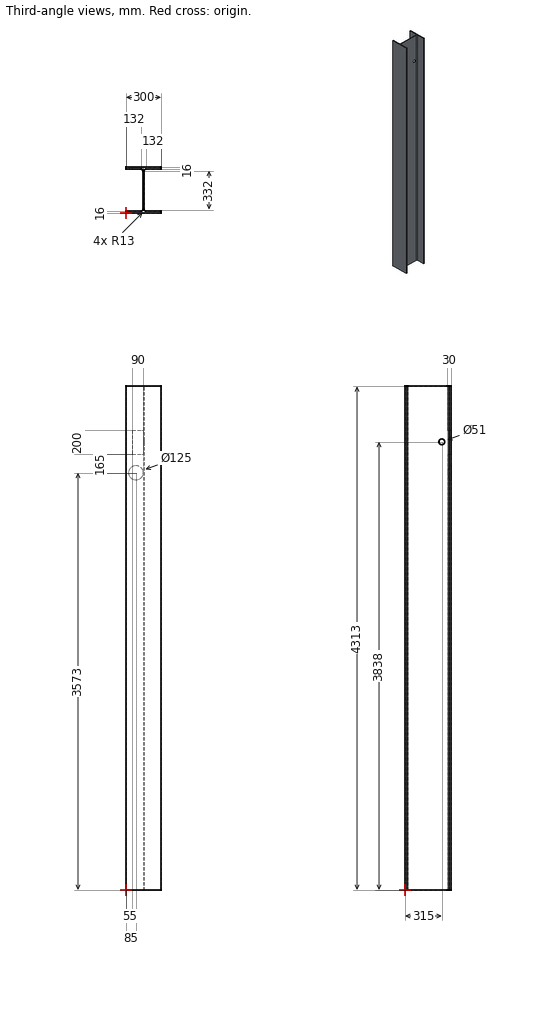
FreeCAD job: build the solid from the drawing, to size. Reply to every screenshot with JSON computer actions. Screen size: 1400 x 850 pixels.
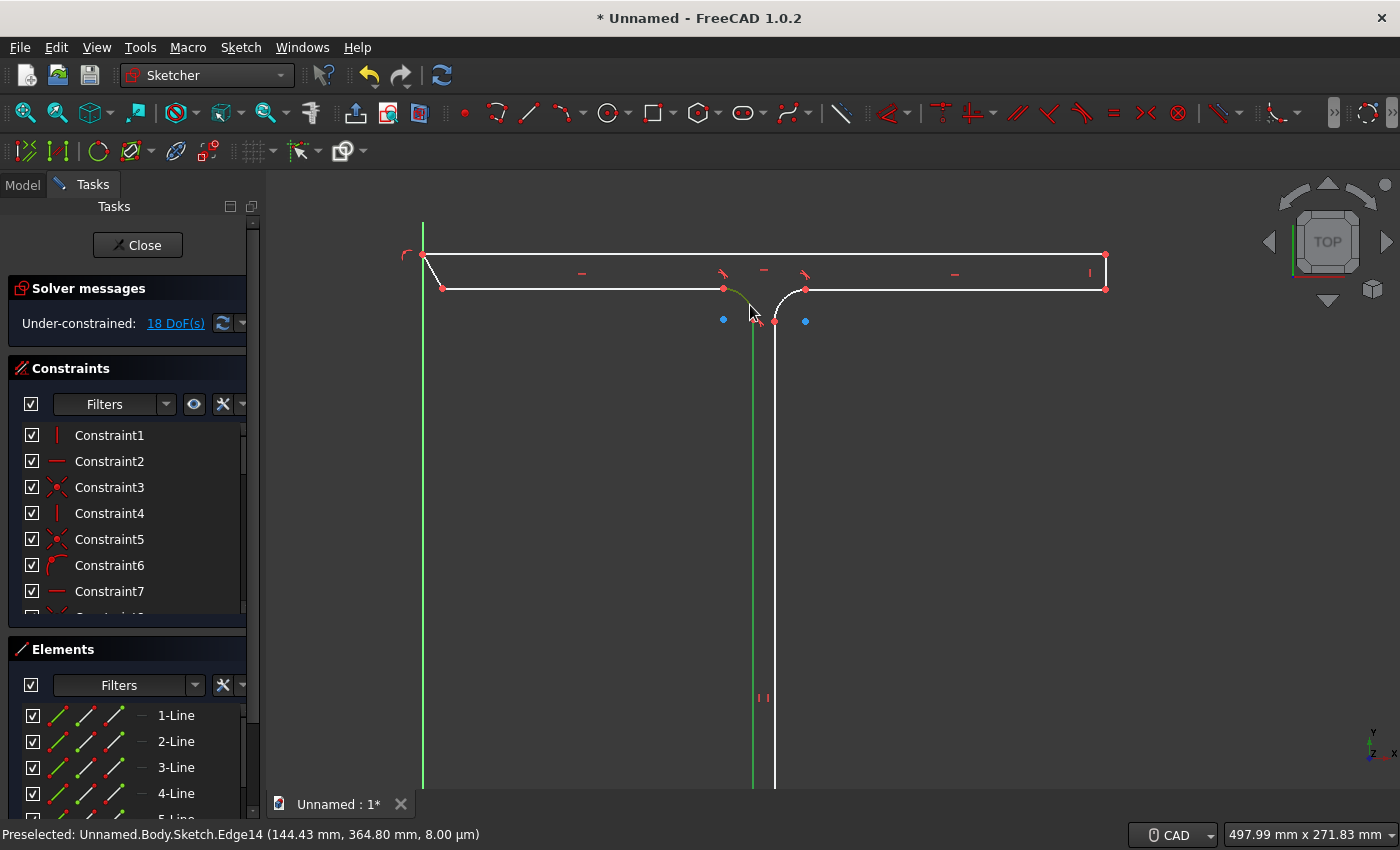
{"action": "left_click", "coordinate": [1082, 114]}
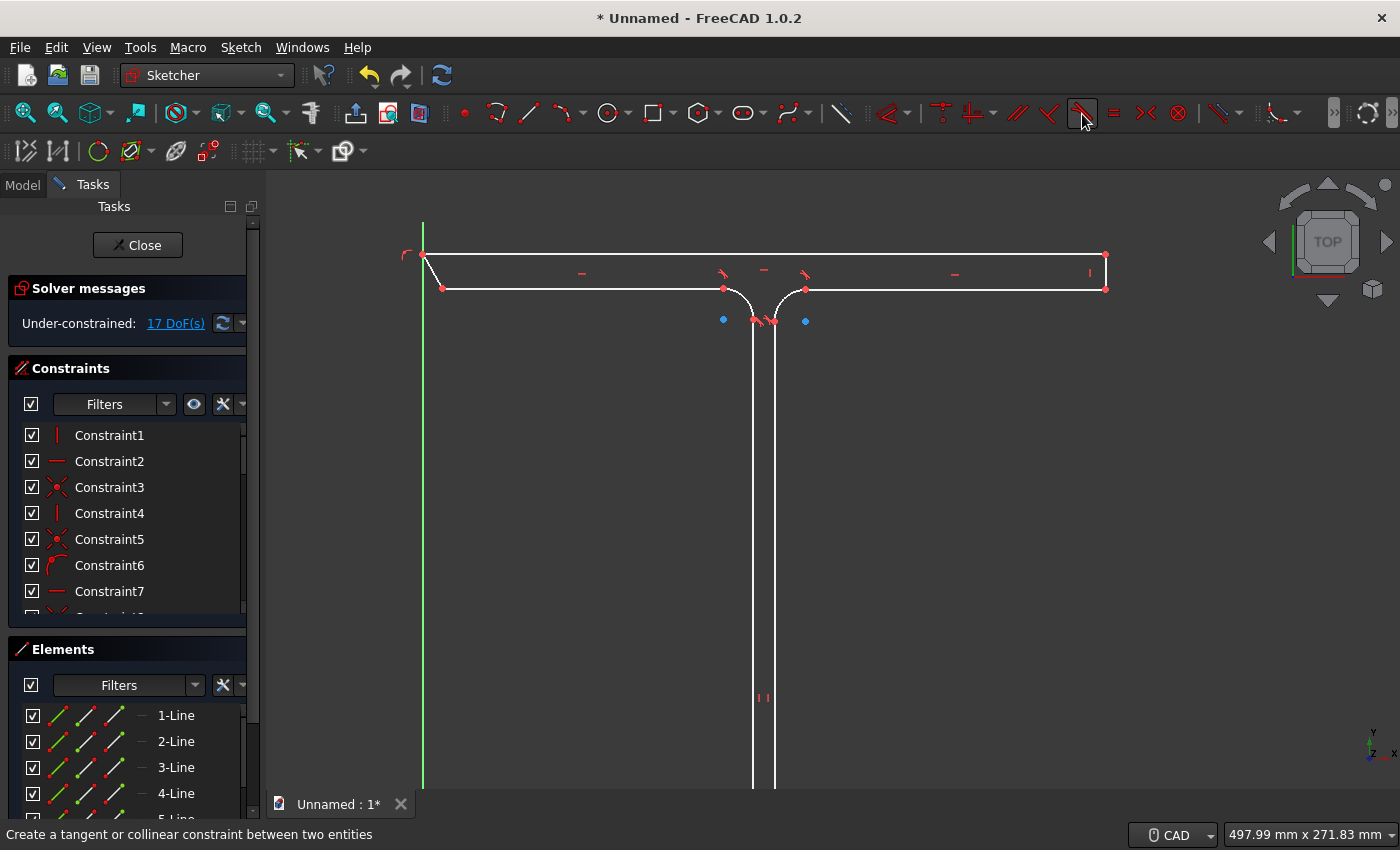
{"action": "left_click", "coordinate": [753, 546]}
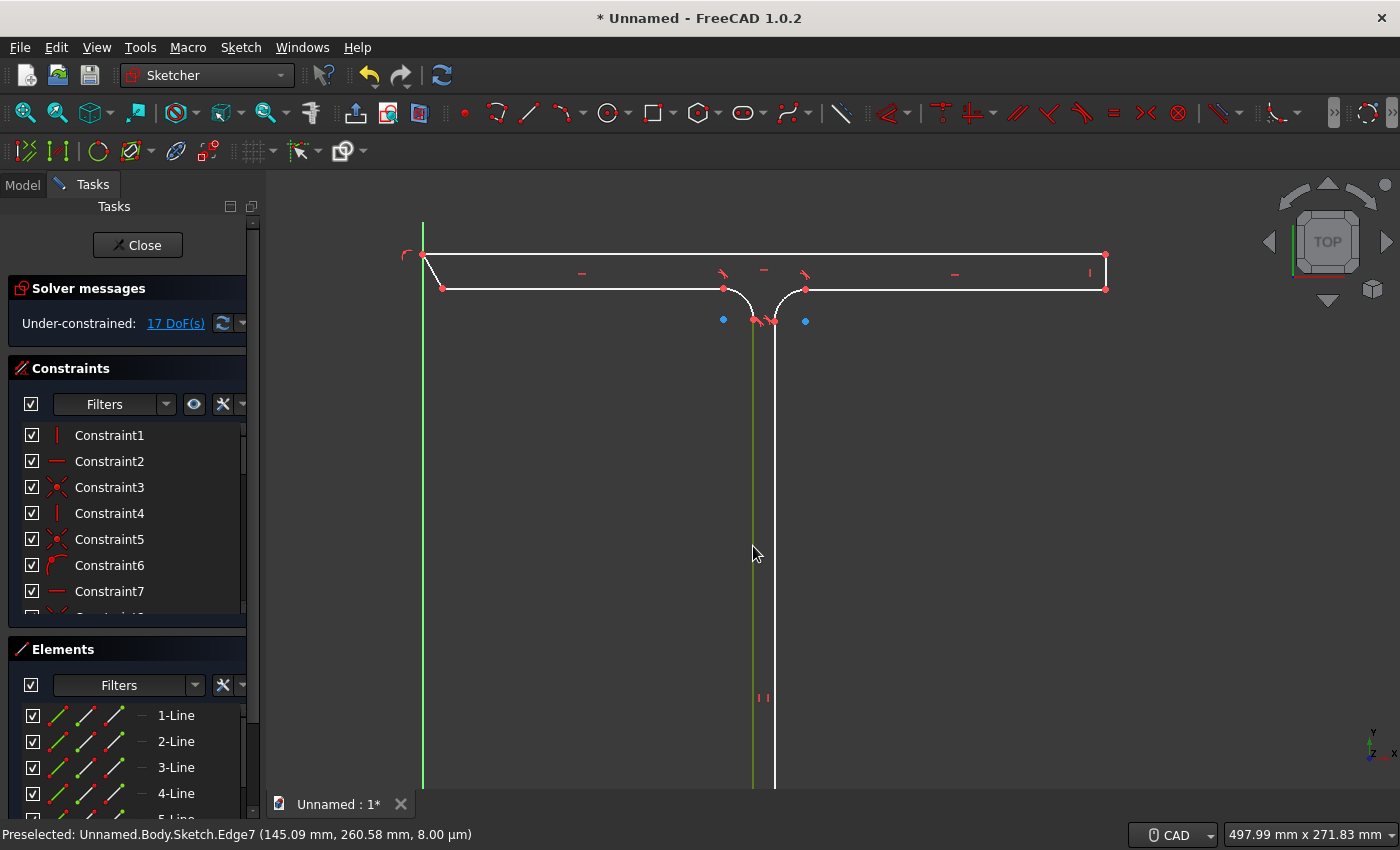
{"action": "scroll", "coordinate": [764, 303], "scroll_direction": "down", "scroll_amount": 4}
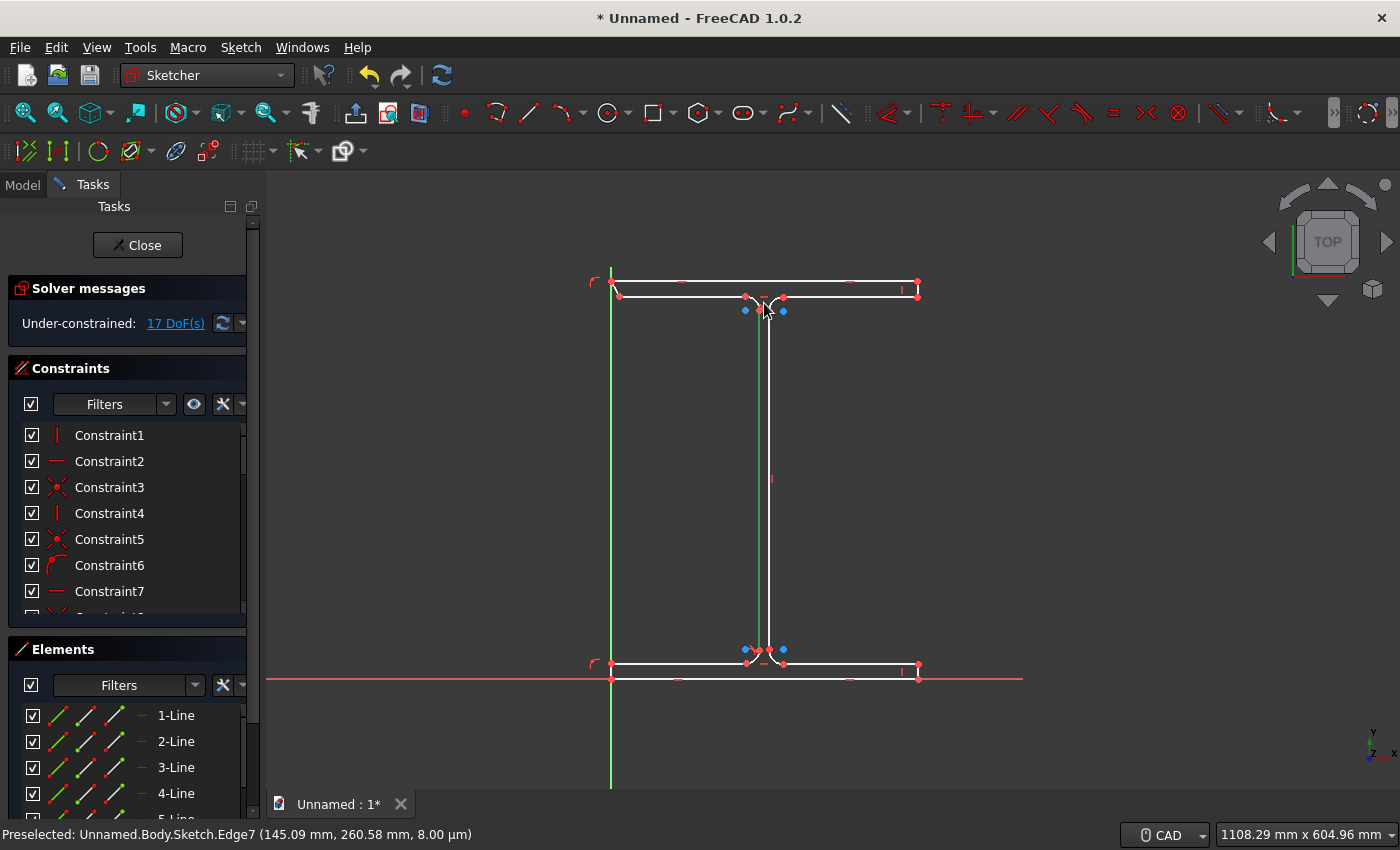
{"action": "scroll", "coordinate": [752, 662], "scroll_direction": "up", "scroll_amount": 5}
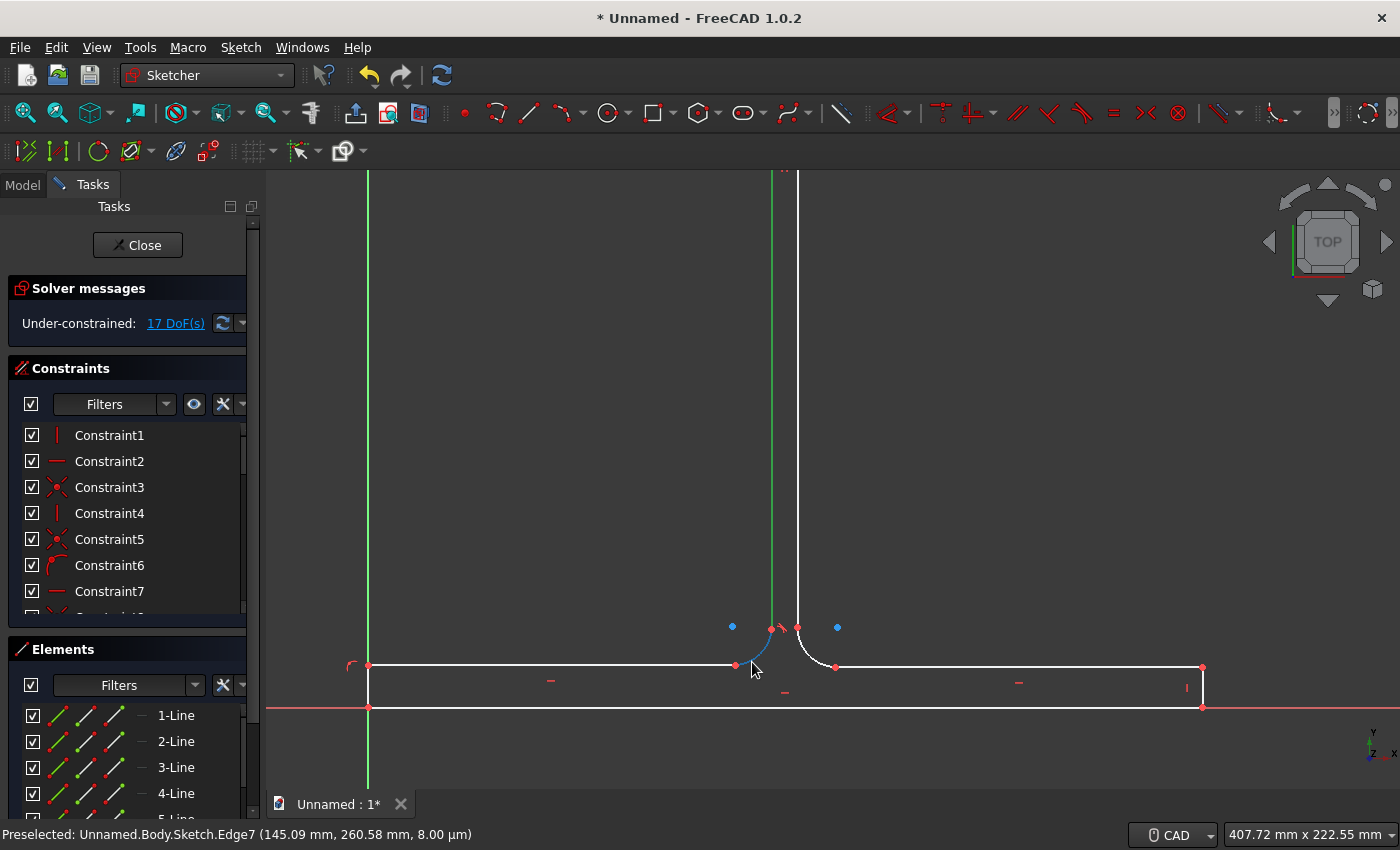
{"action": "left_click", "coordinate": [751, 660]}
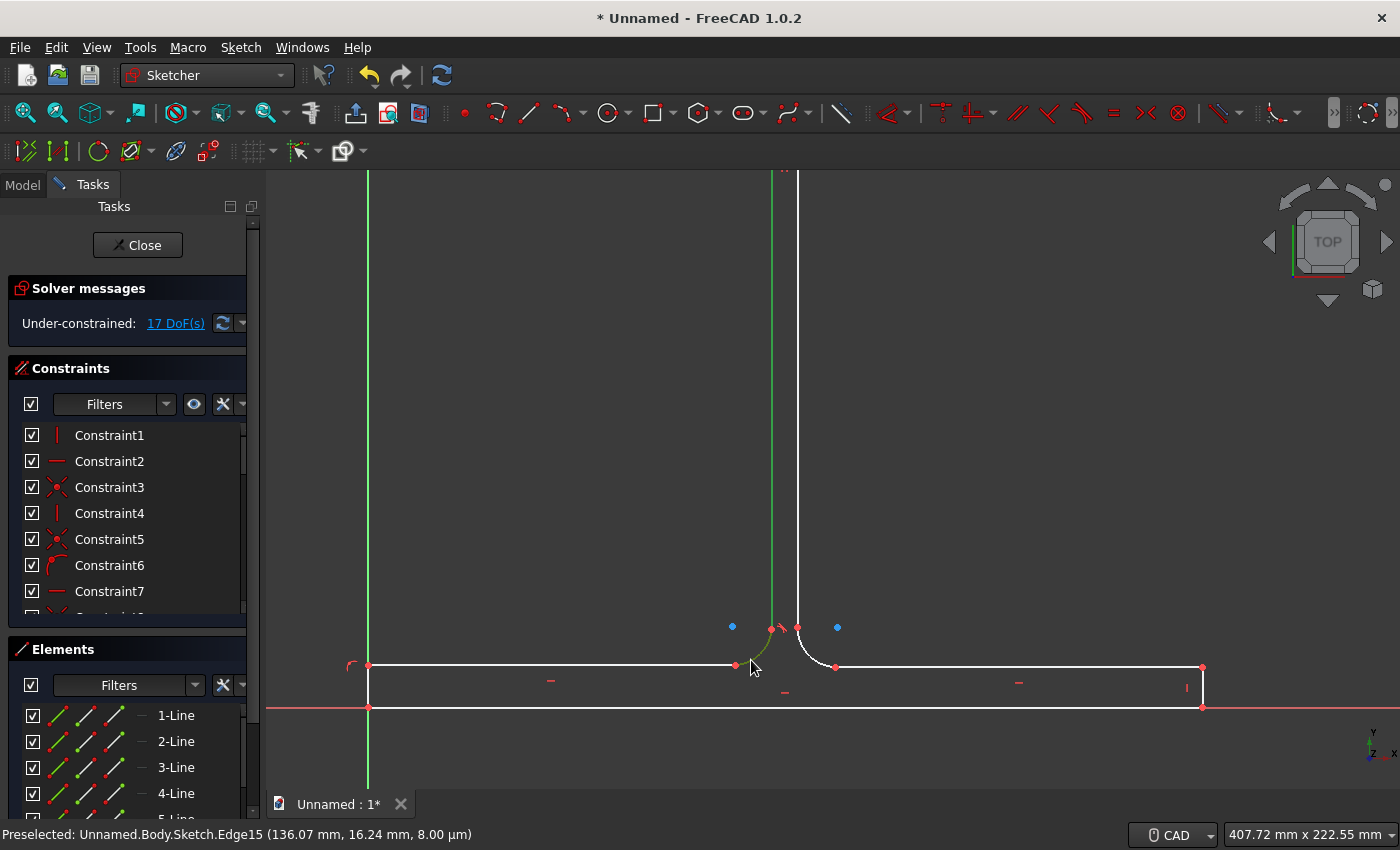
{"action": "left_click", "coordinate": [1082, 114]}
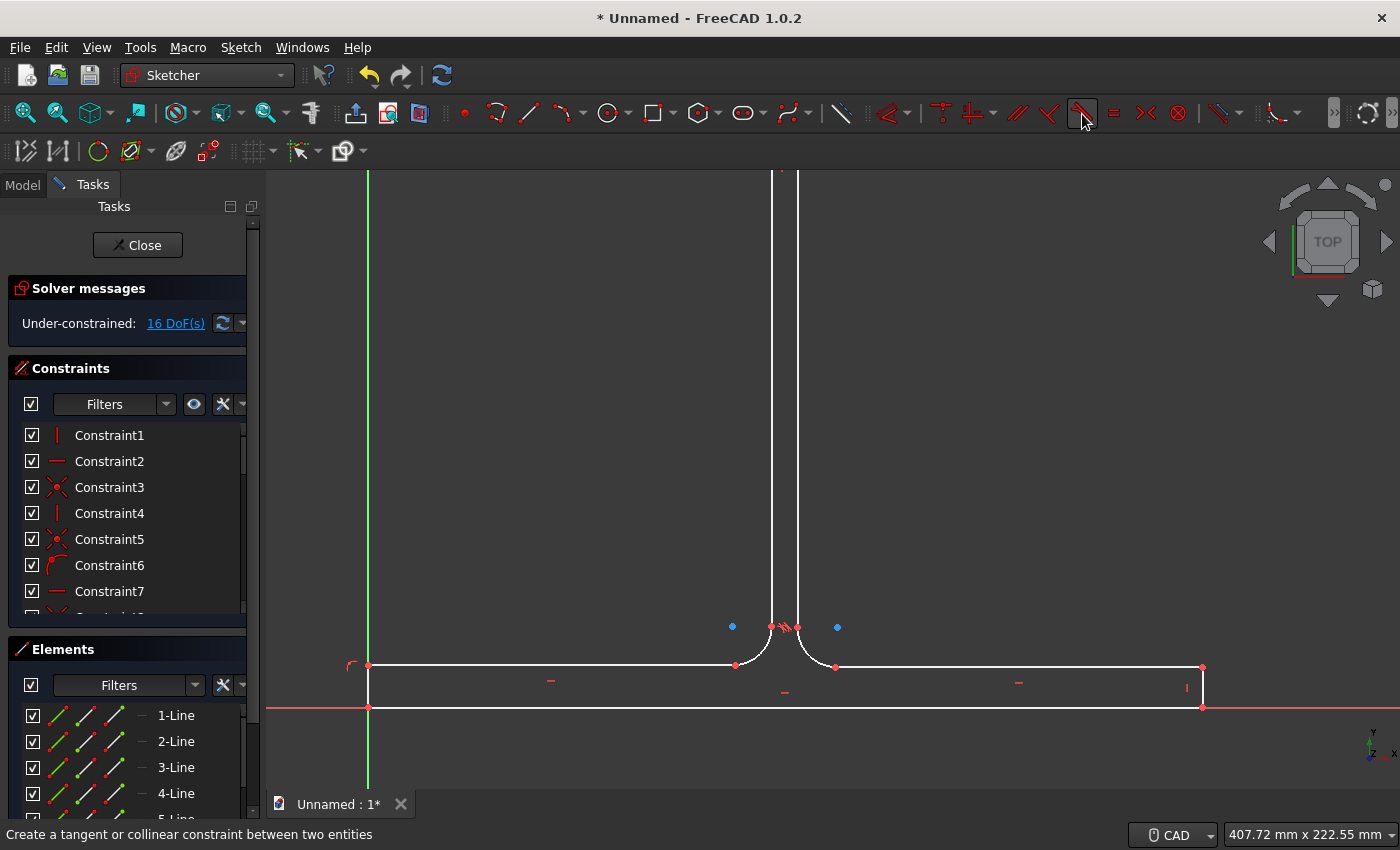
{"action": "left_click", "coordinate": [625, 665]}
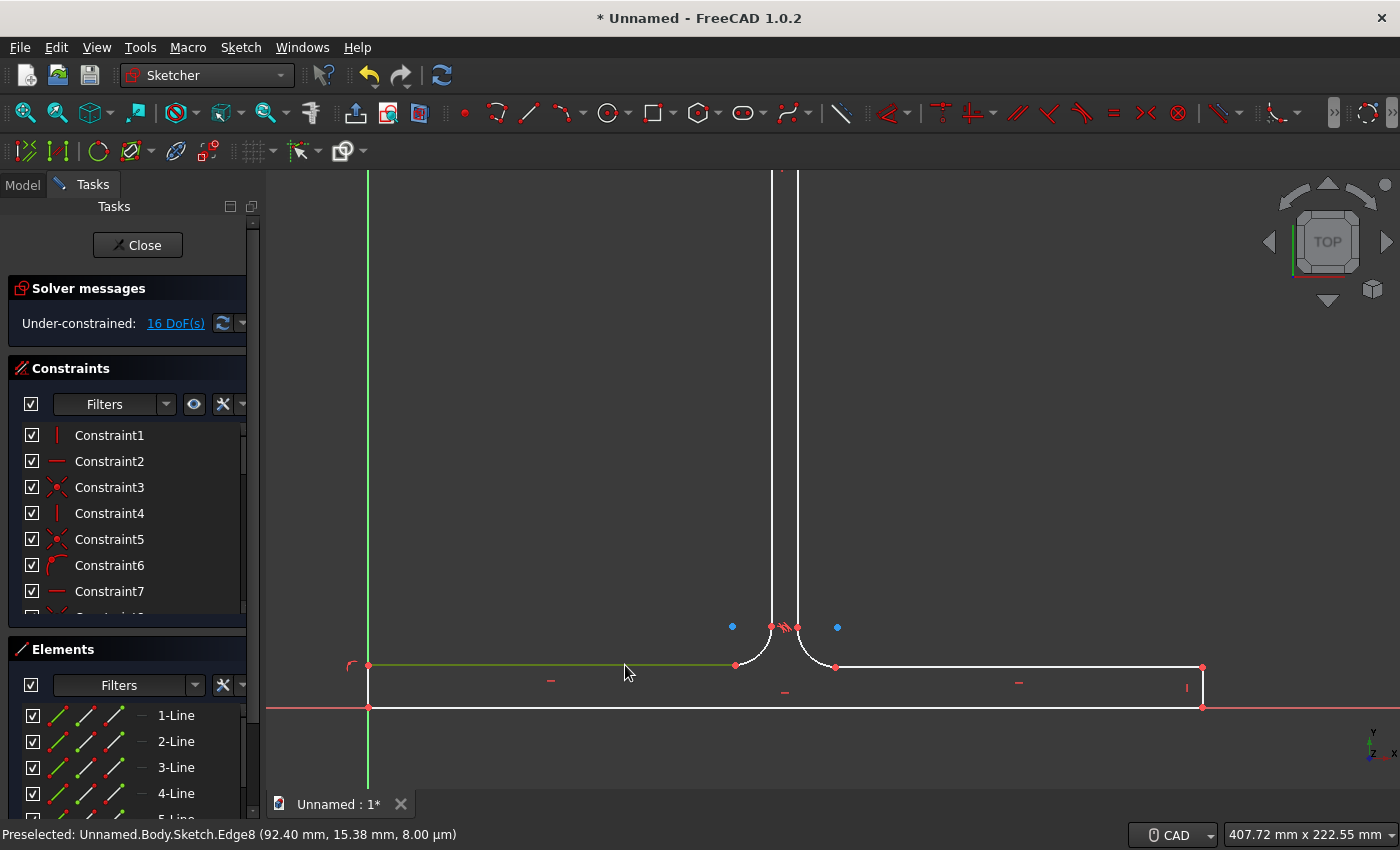
{"action": "left_click", "coordinate": [752, 660]}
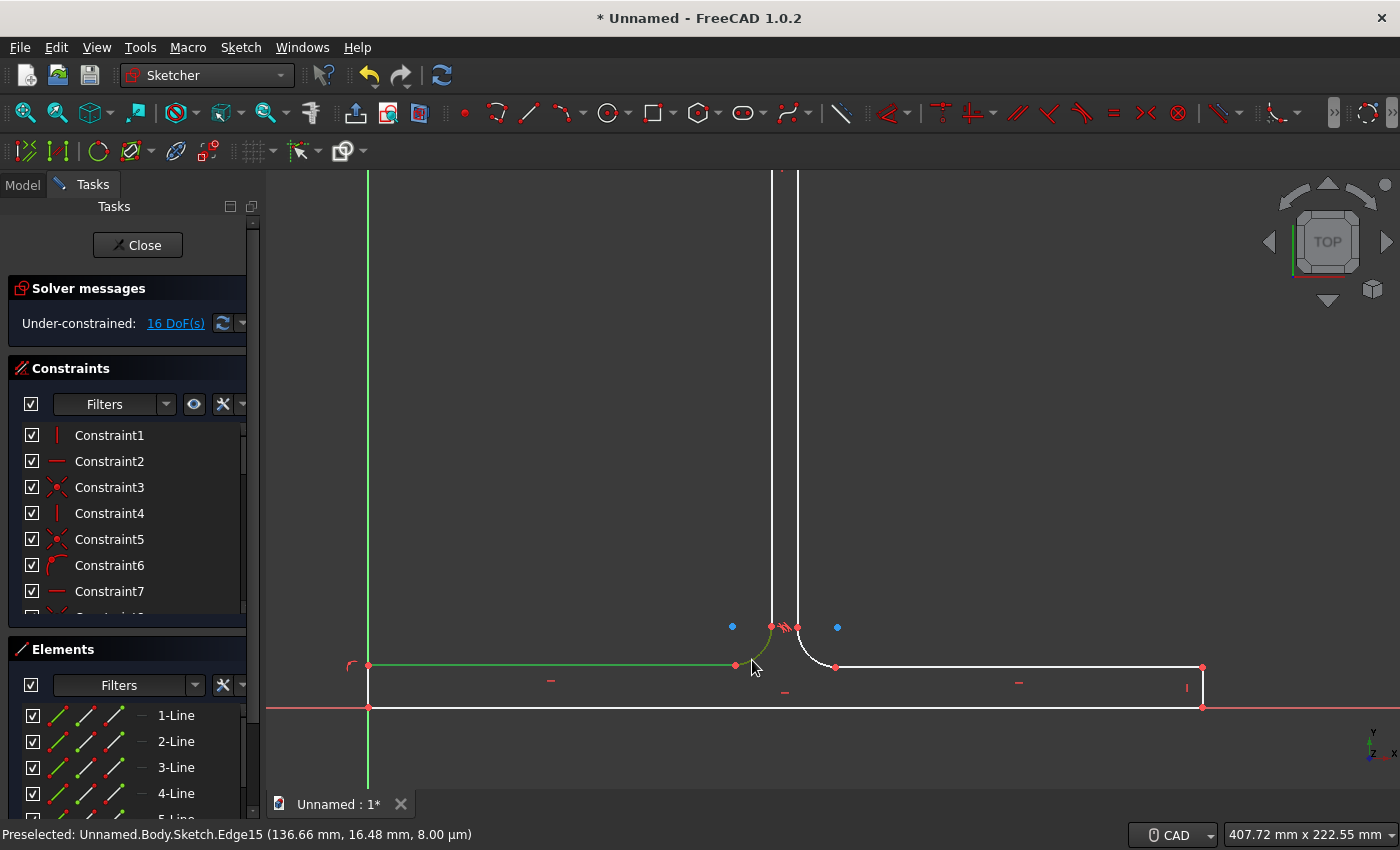
{"action": "left_click", "coordinate": [1082, 114]}